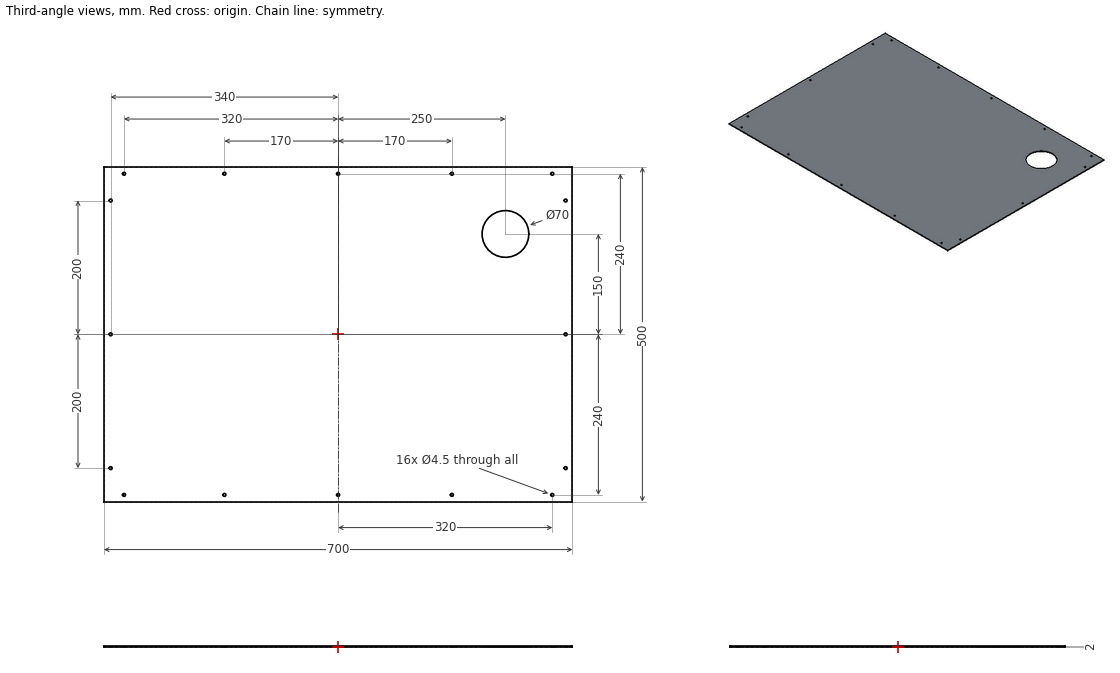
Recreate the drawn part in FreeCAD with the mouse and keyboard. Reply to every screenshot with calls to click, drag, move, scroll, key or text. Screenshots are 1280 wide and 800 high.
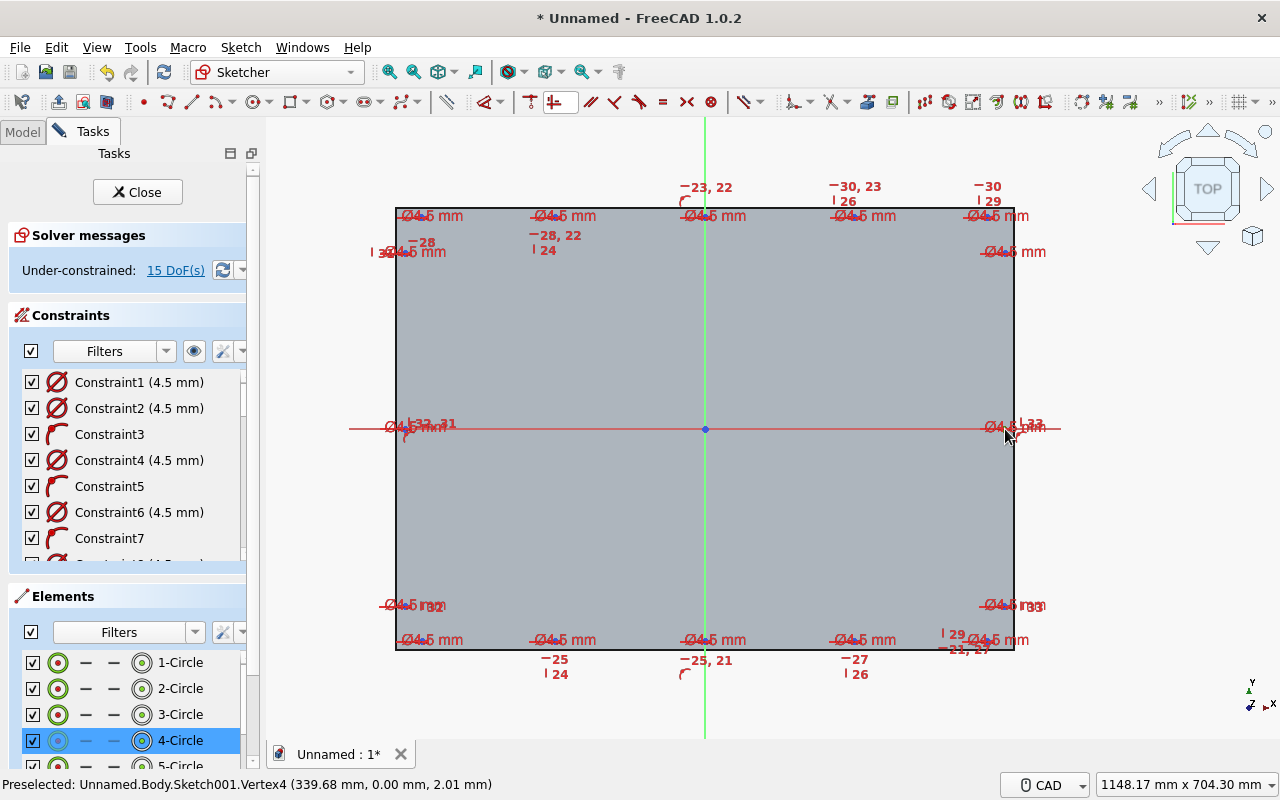
click(1005, 254)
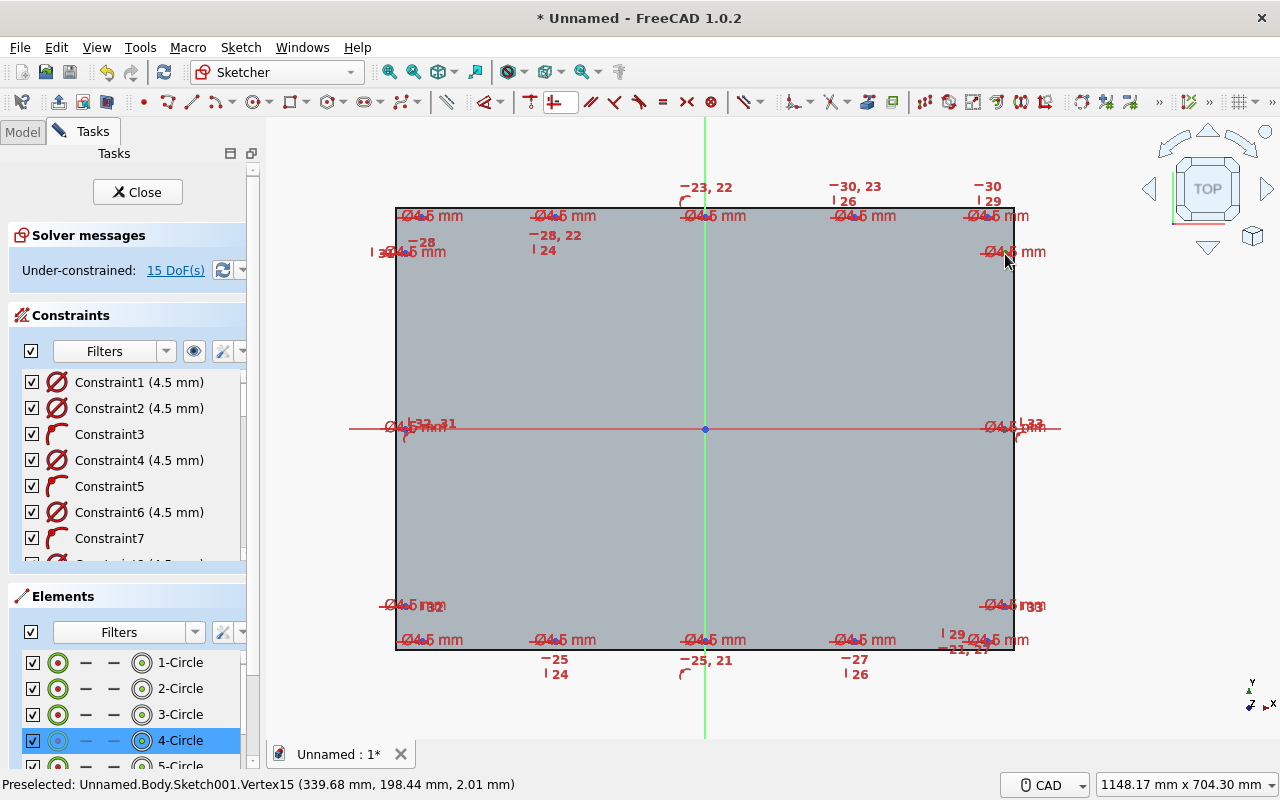
click(572, 102)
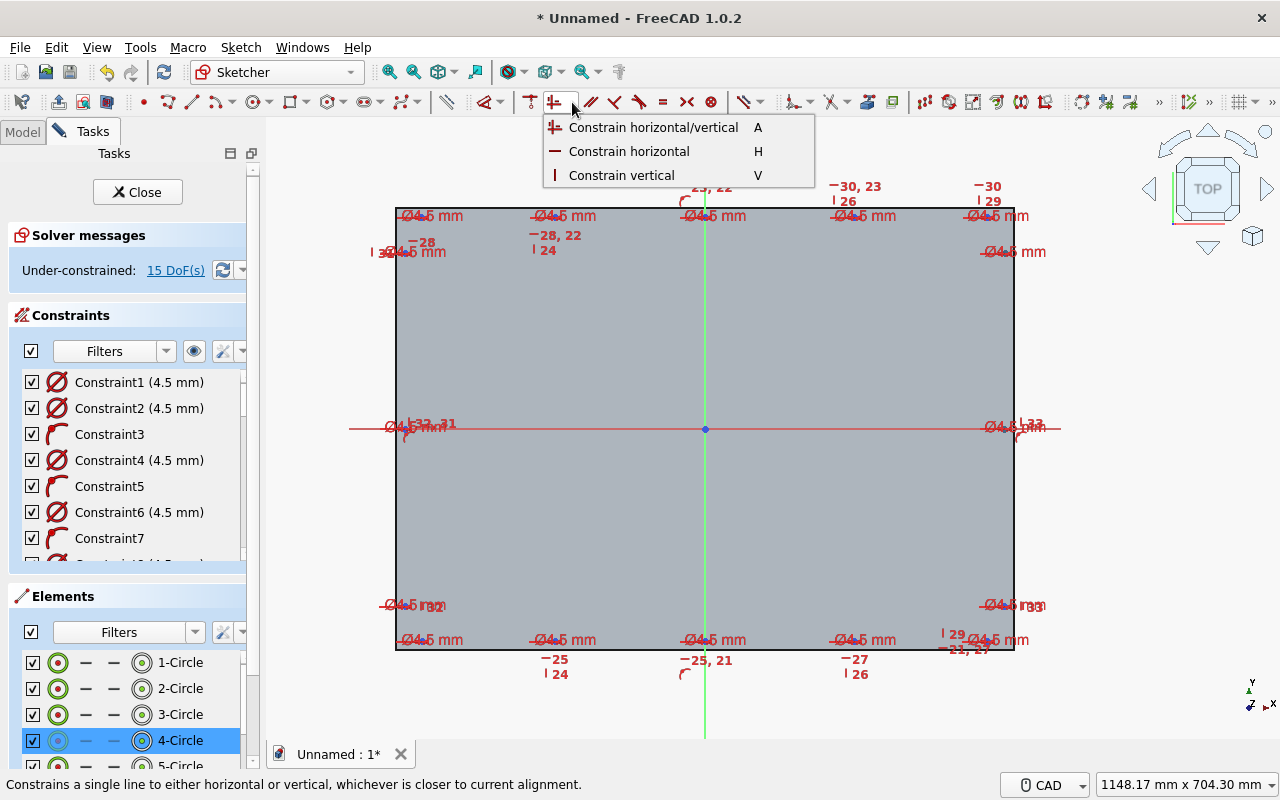
click(679, 175)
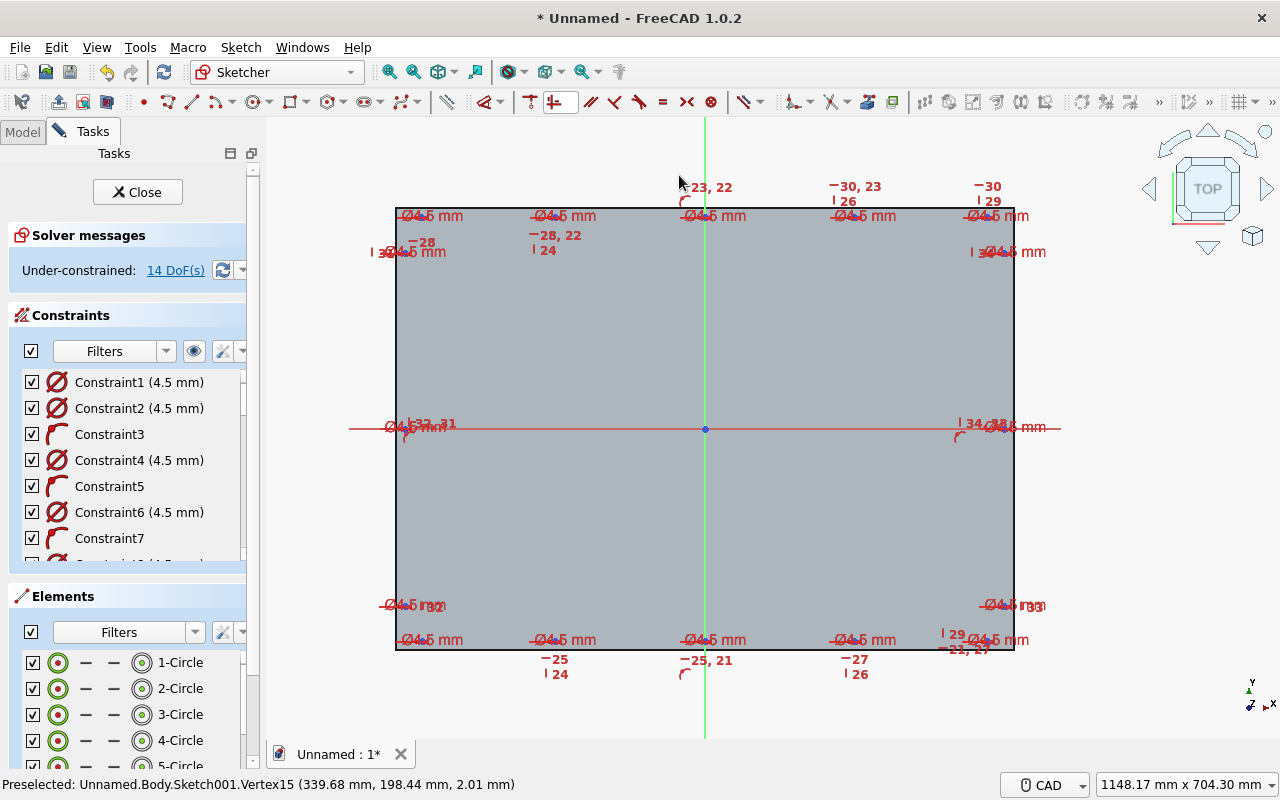
click(422, 218)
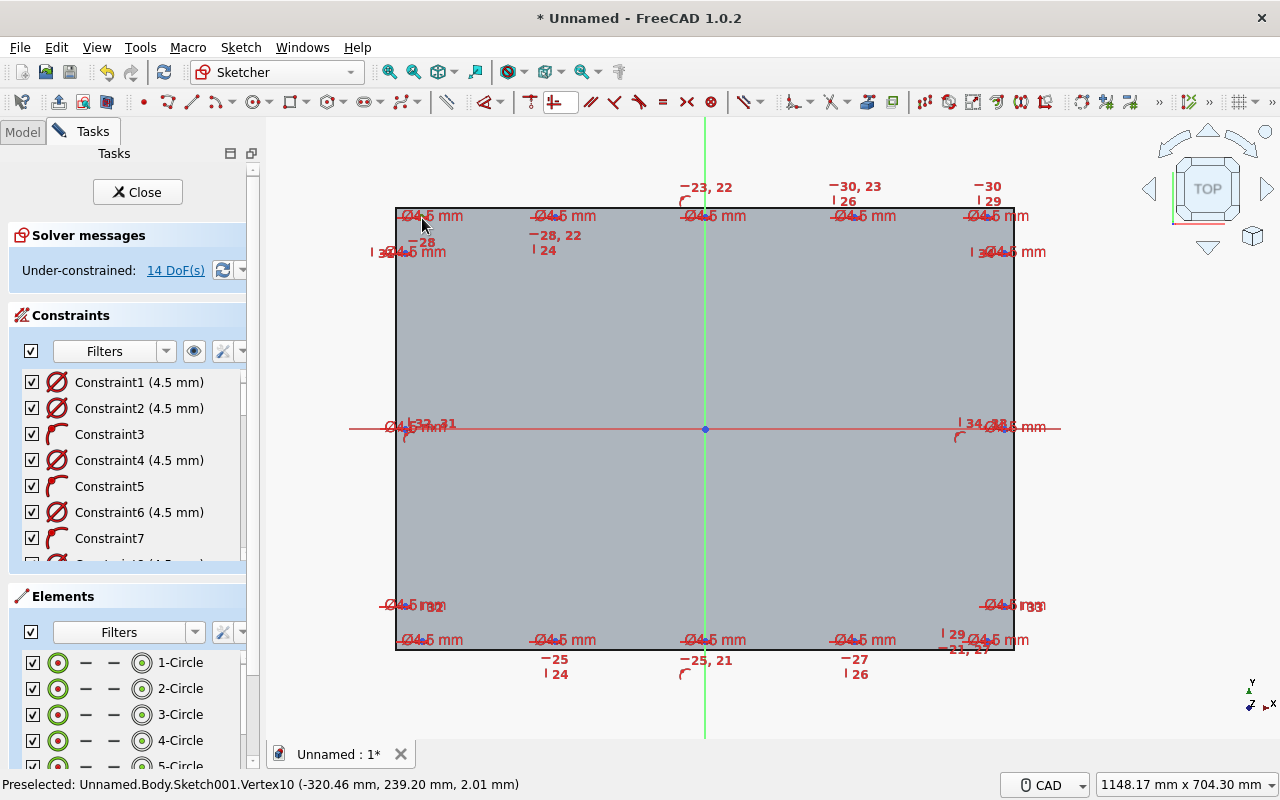
click(422, 642)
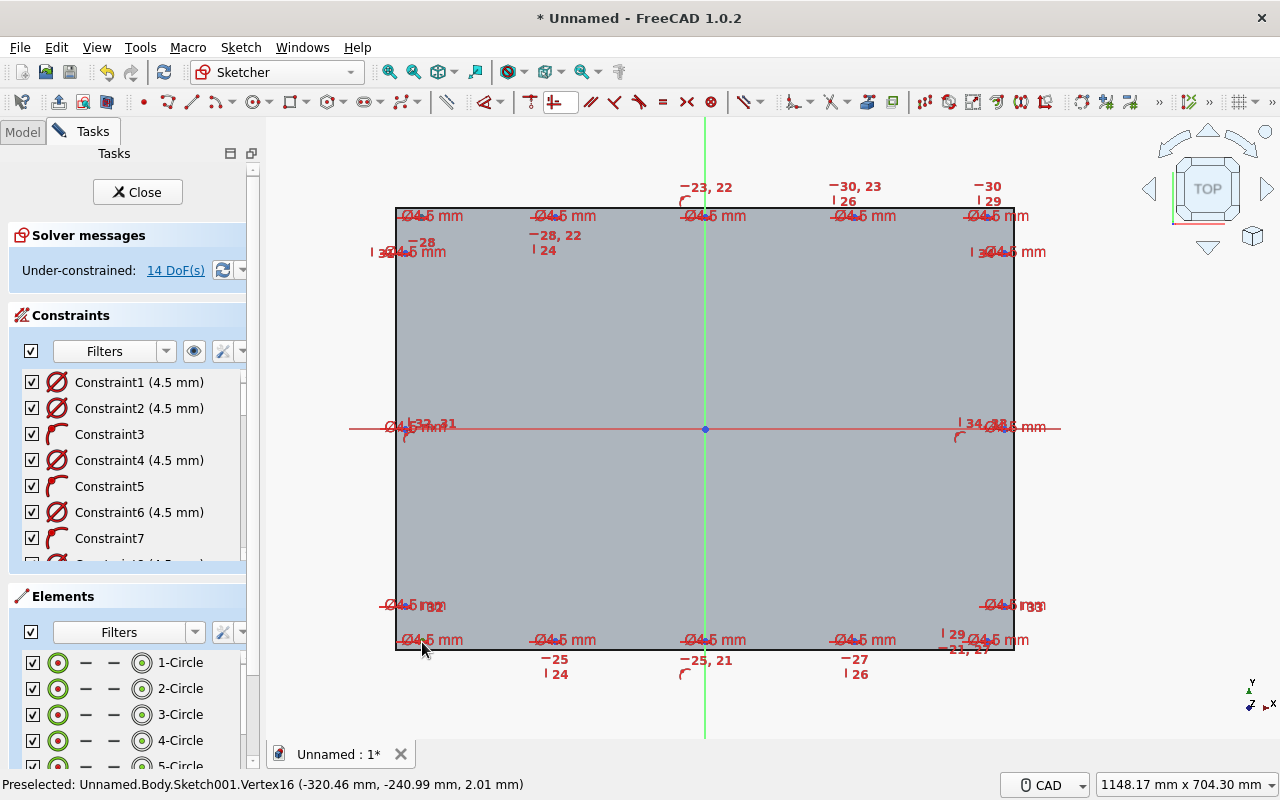
key(v)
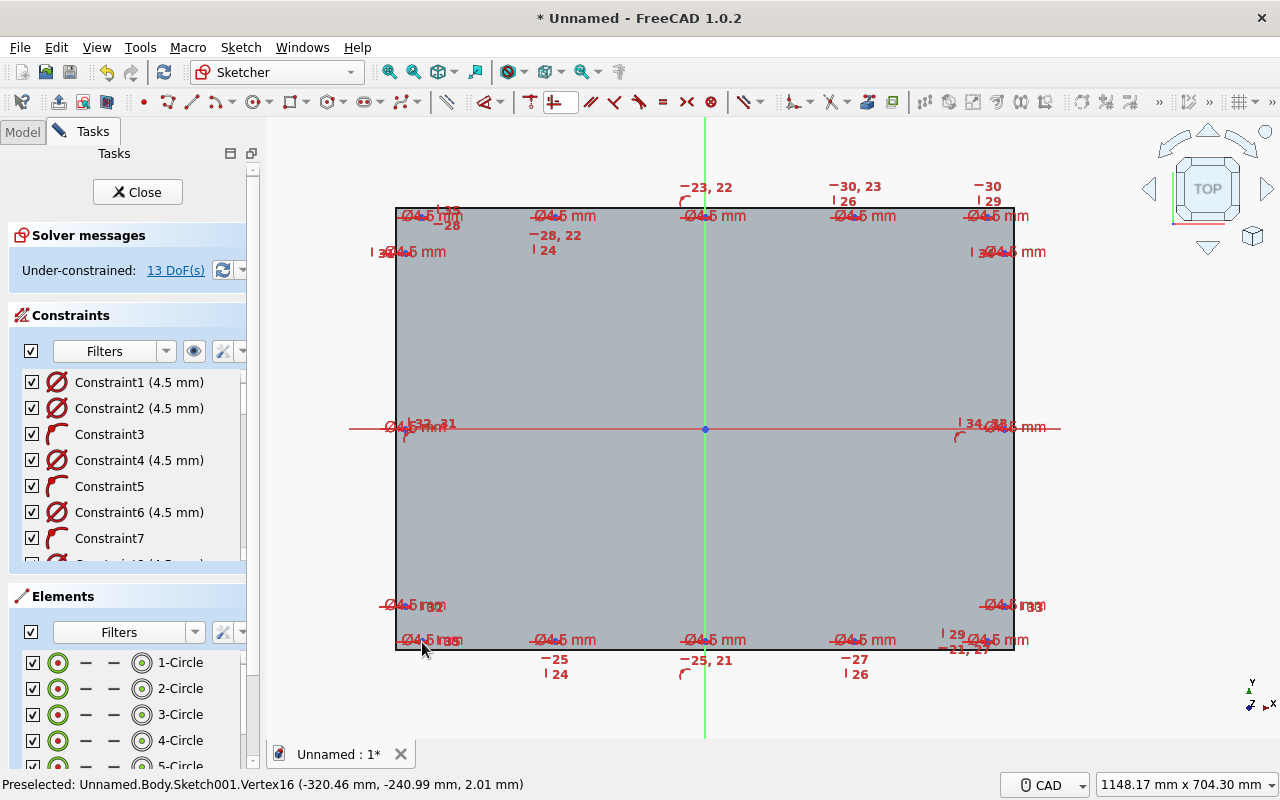
click(555, 642)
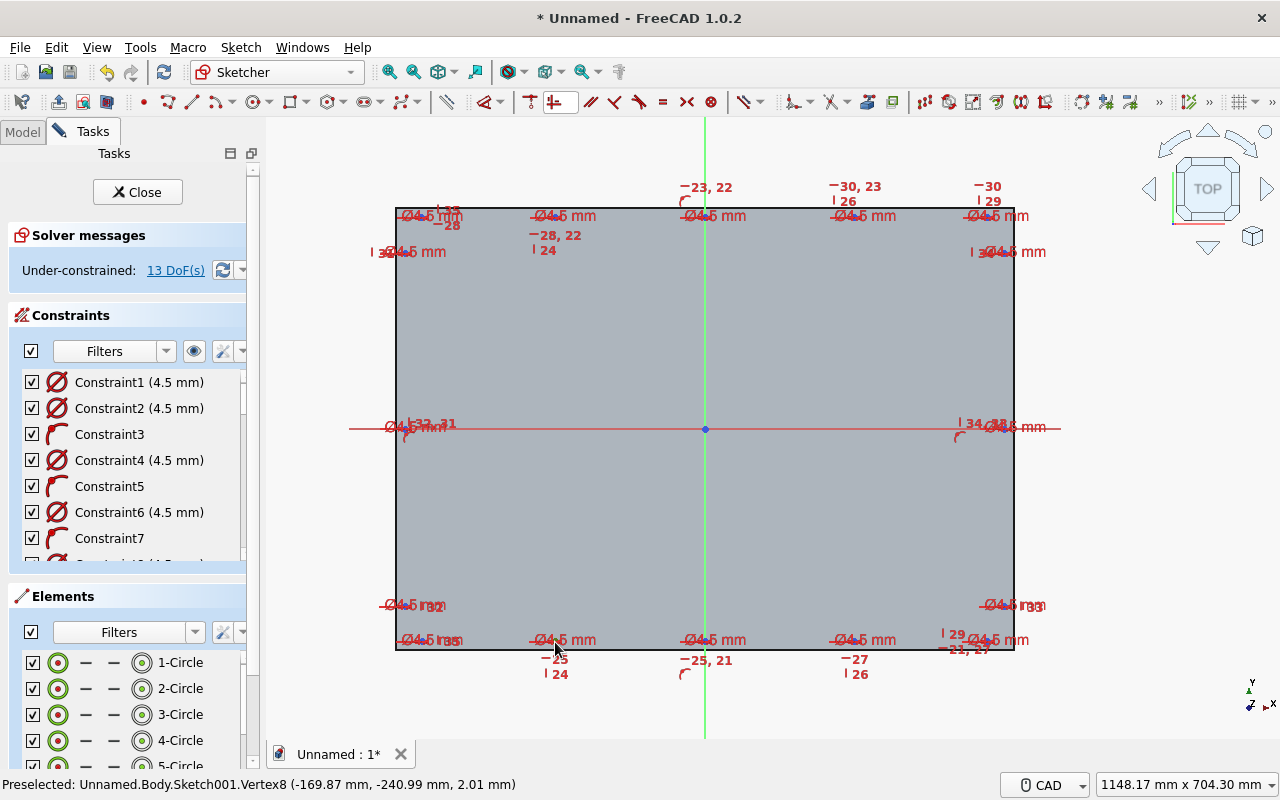
click(422, 642)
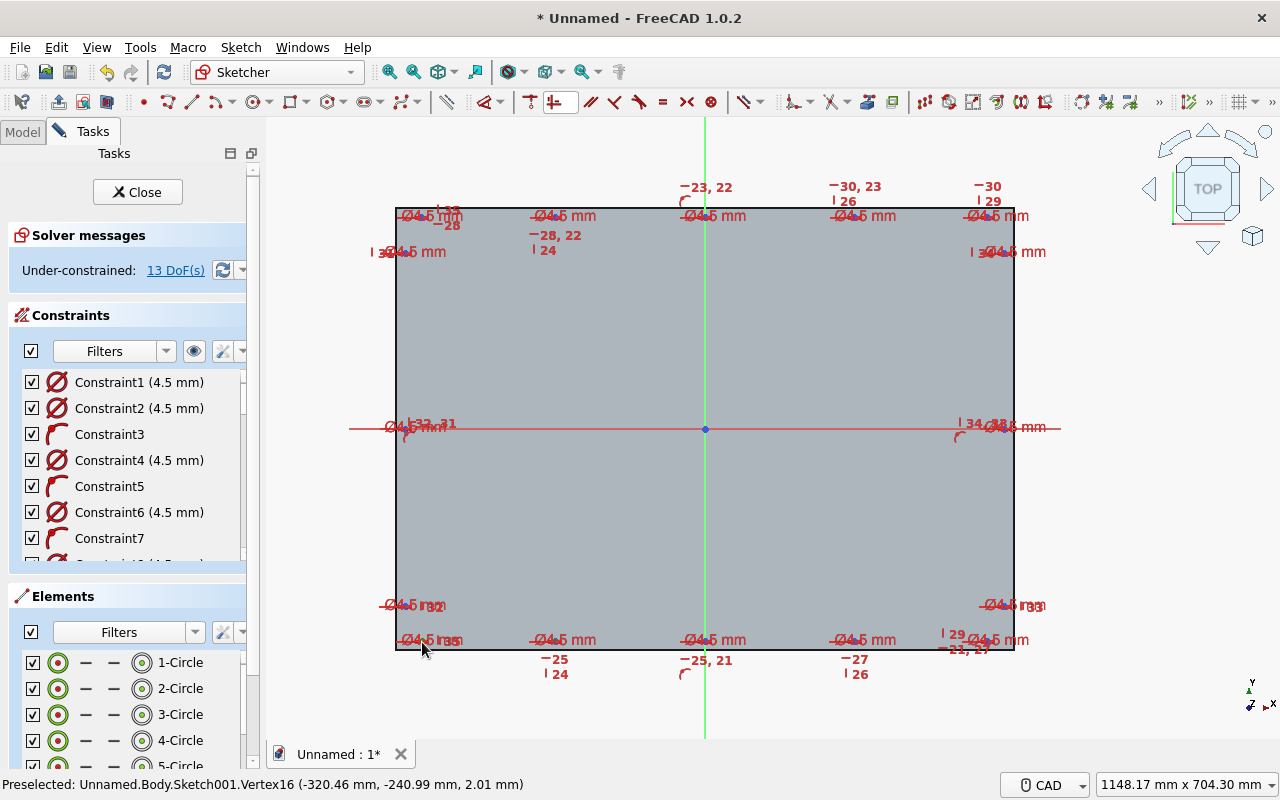
key(h)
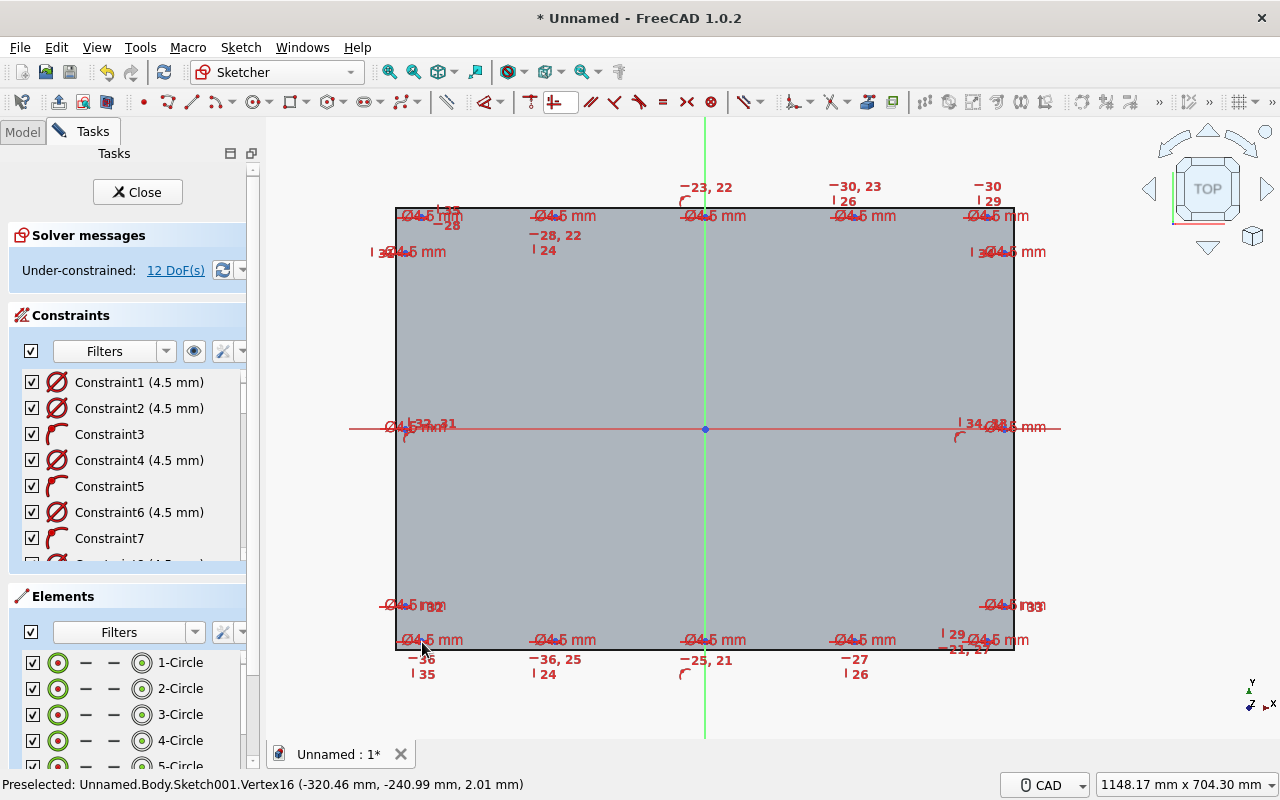
click(405, 607)